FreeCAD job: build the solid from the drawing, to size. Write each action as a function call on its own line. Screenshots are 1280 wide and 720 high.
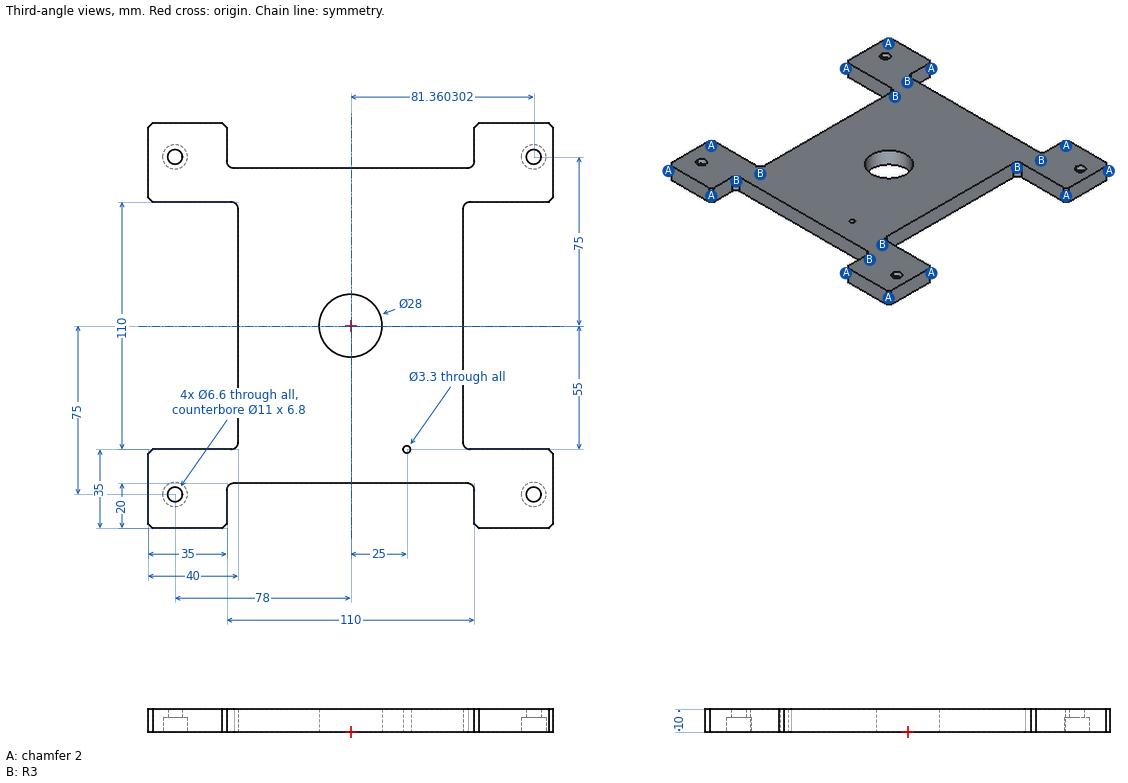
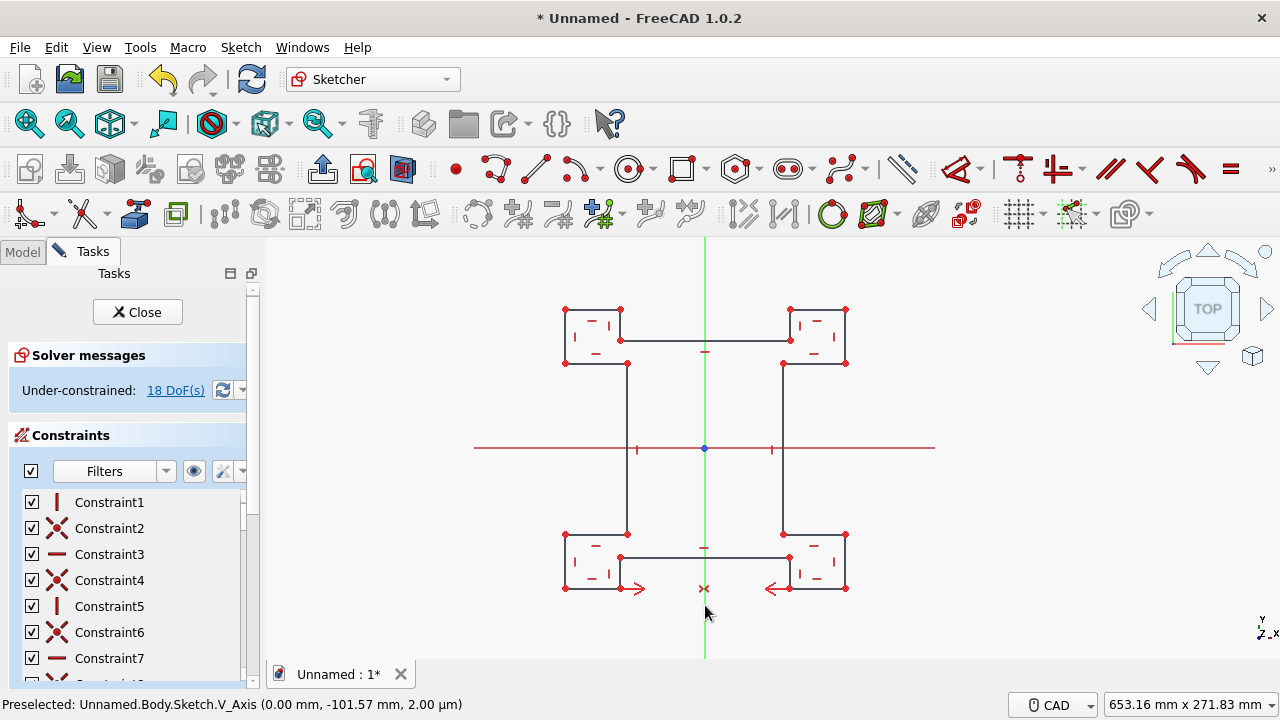
click(565, 535)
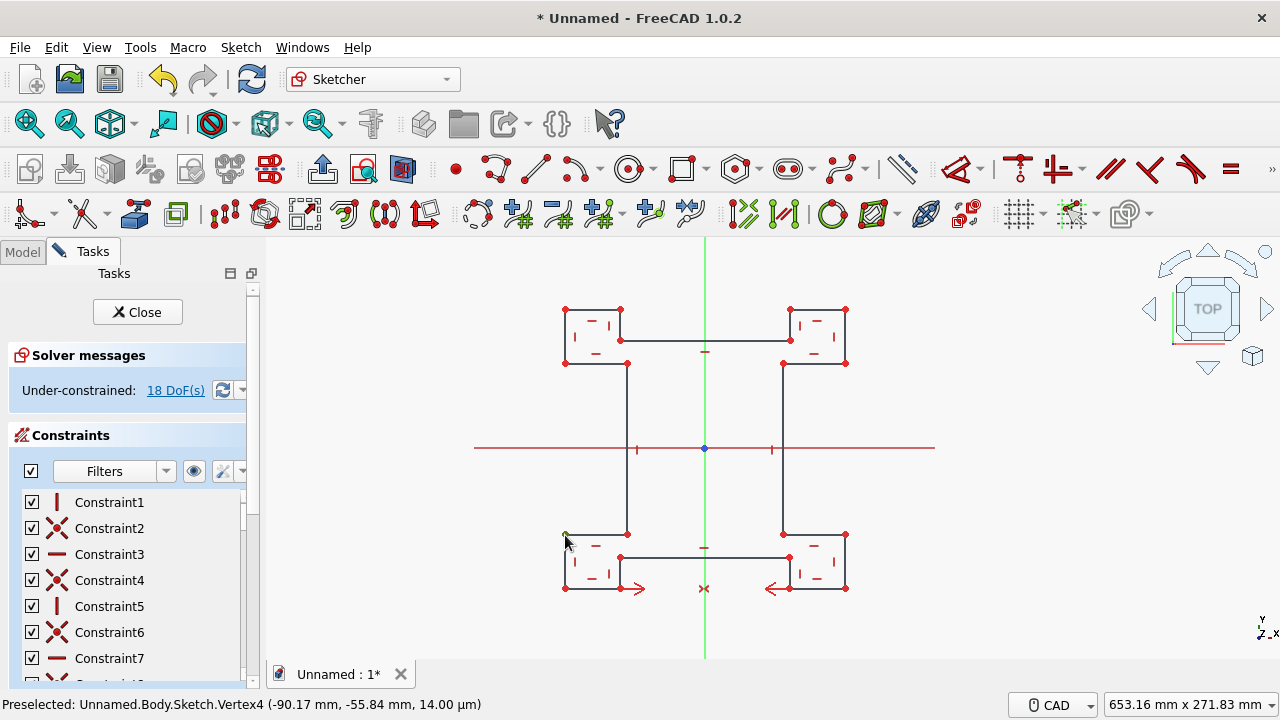
click(845, 535)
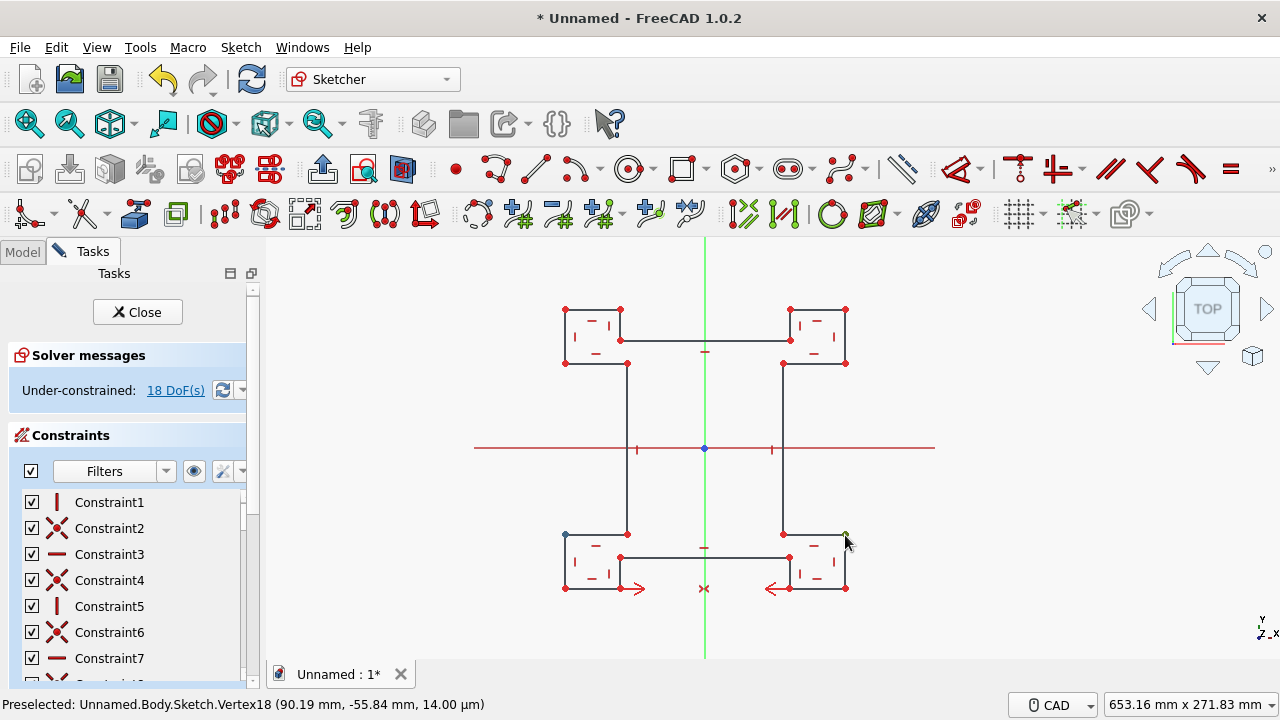
click(705, 605)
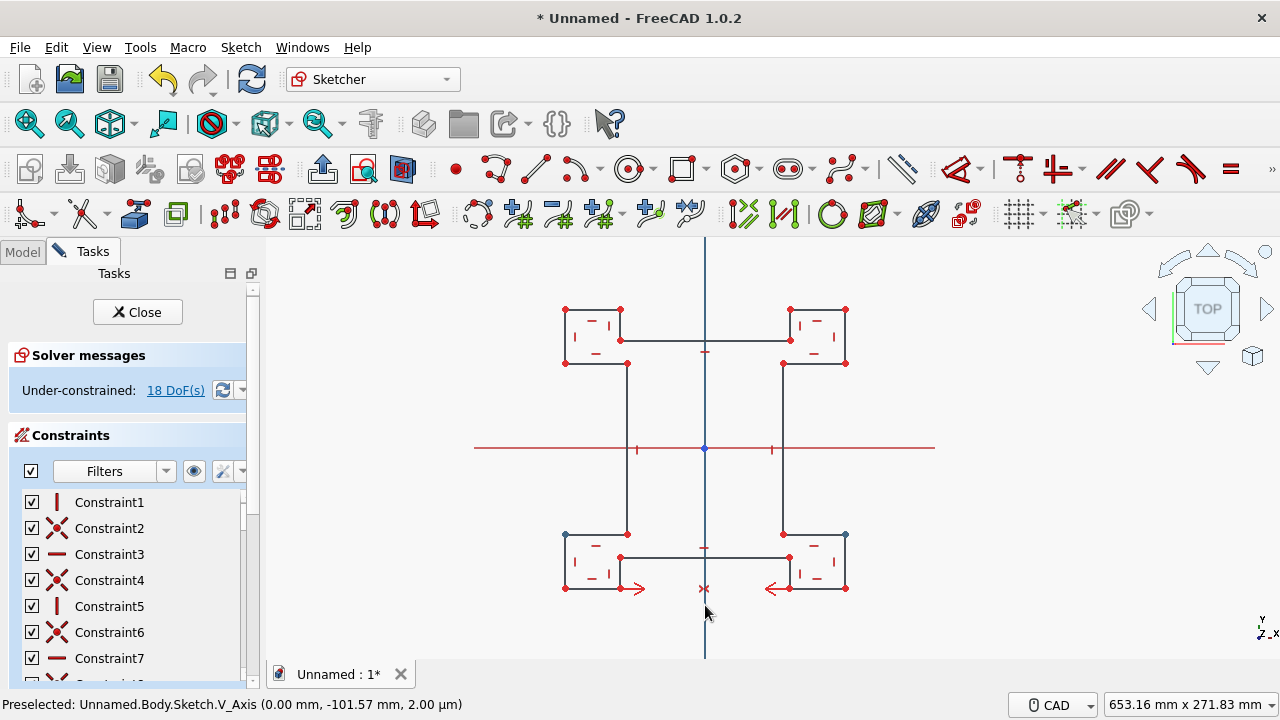
key(s)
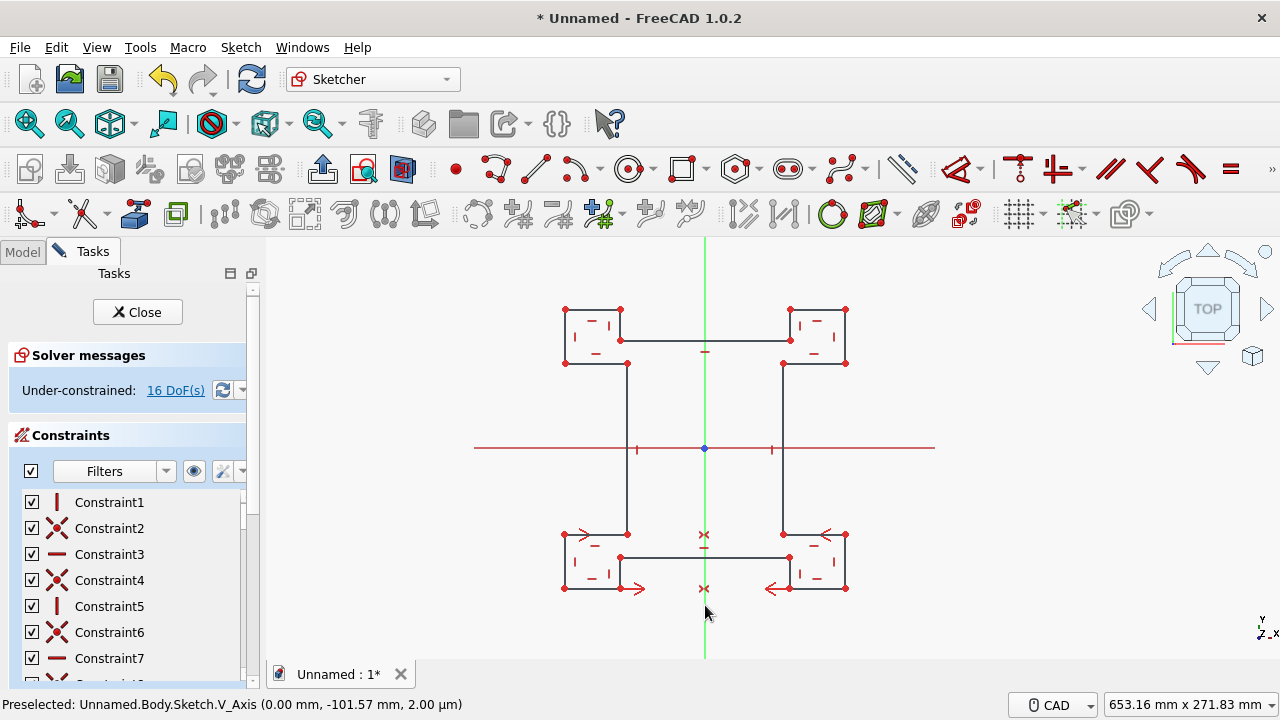
click(627, 364)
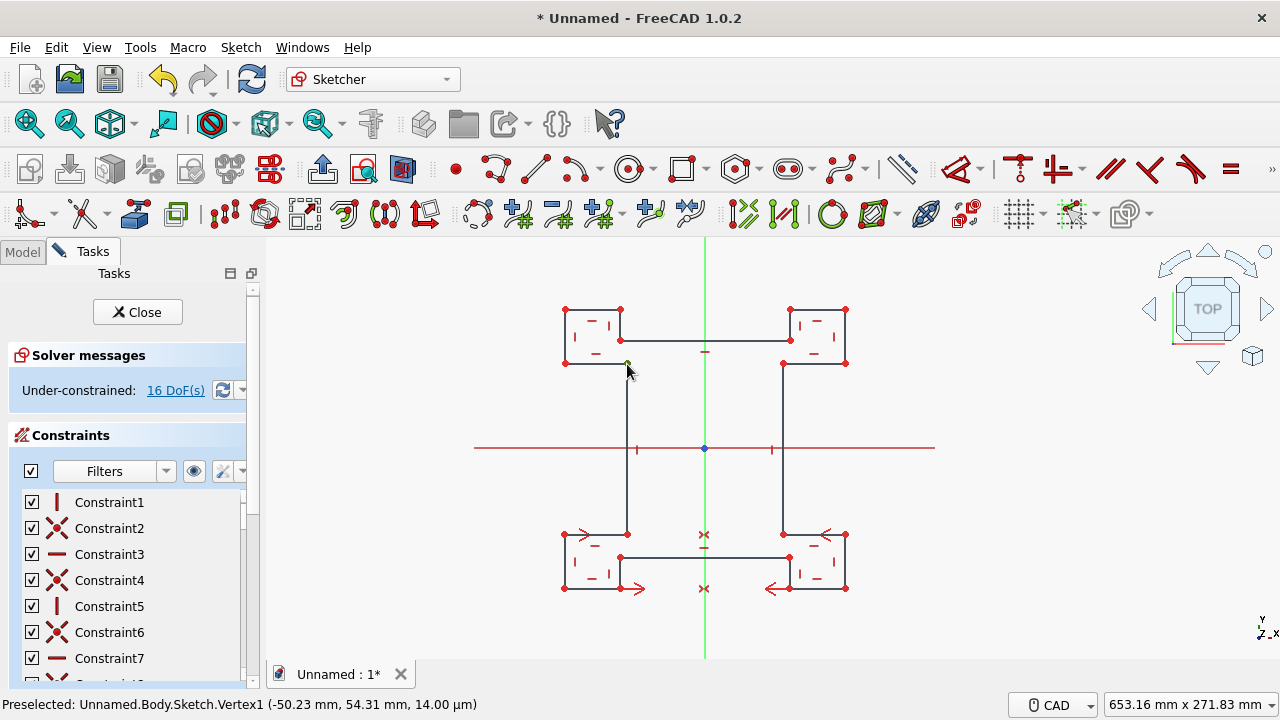
click(783, 364)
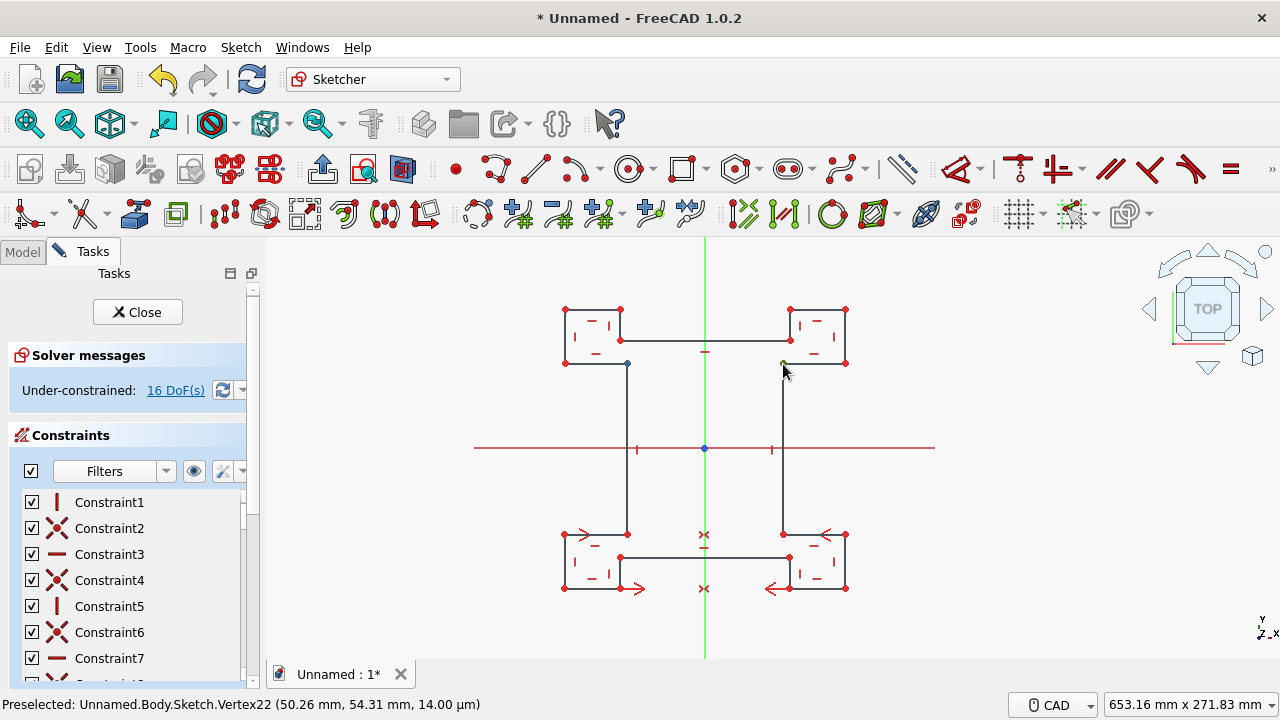
click(705, 605)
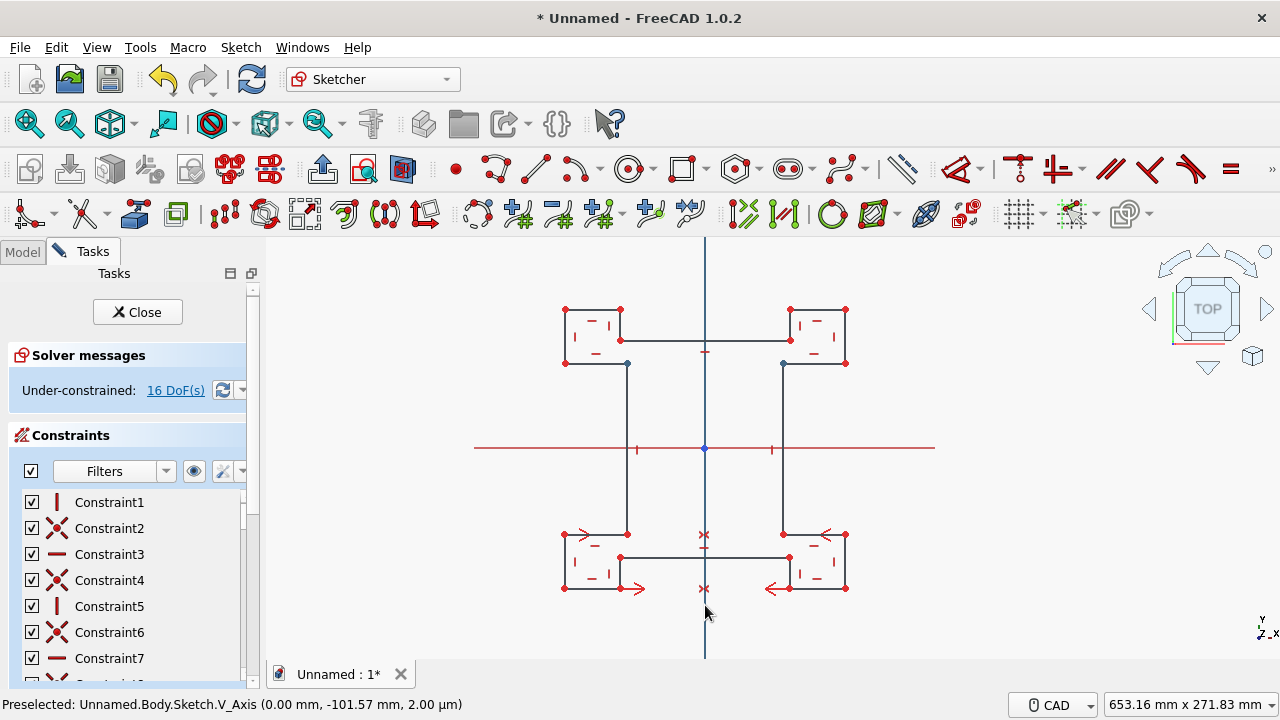
key(s)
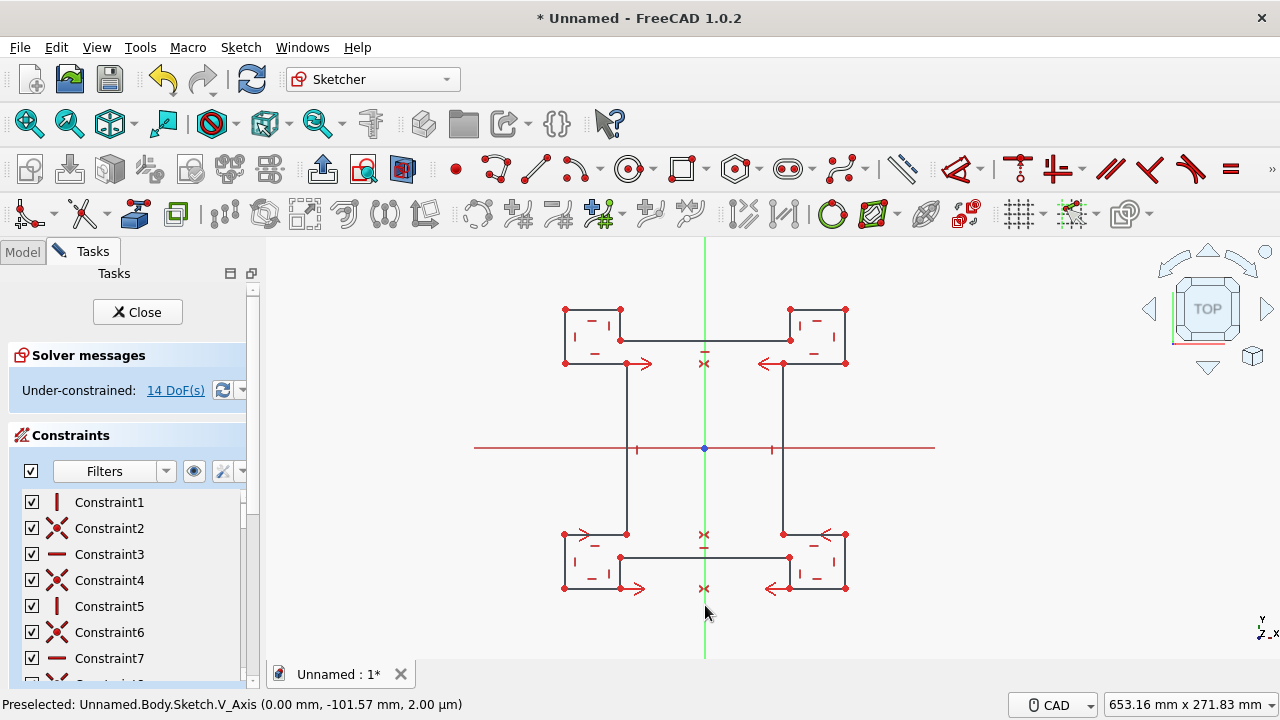
click(845, 535)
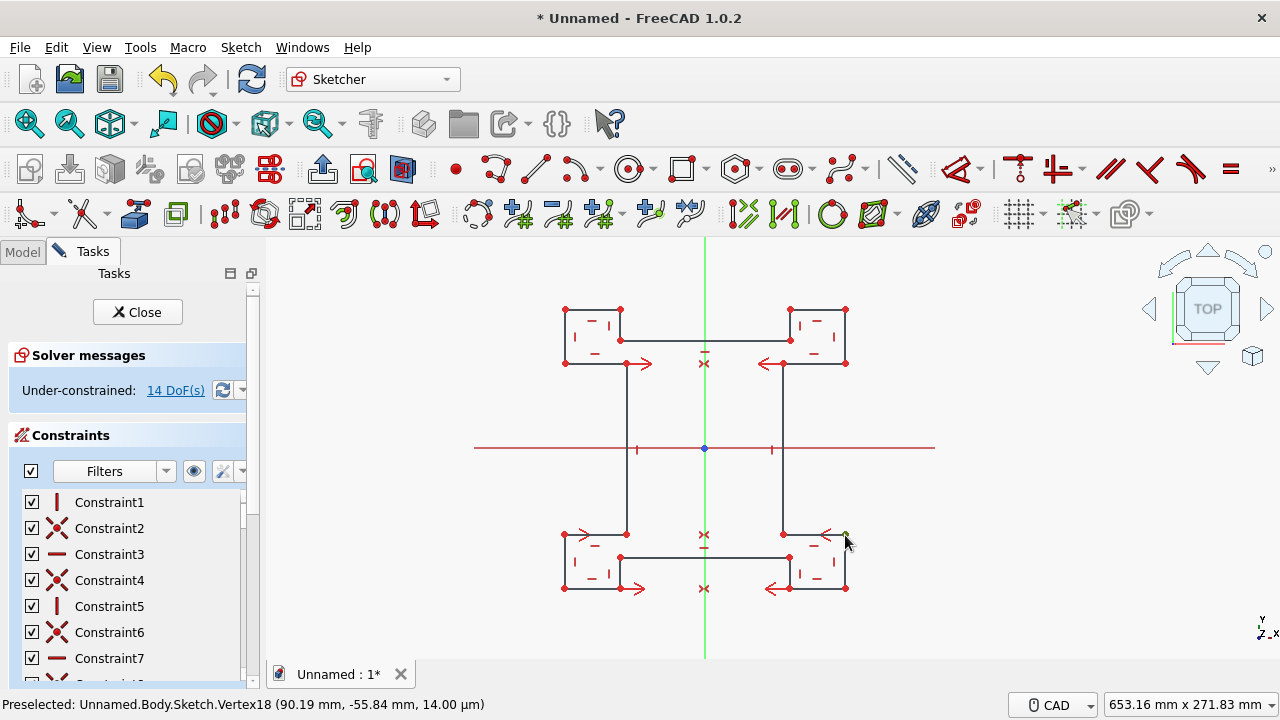
click(845, 364)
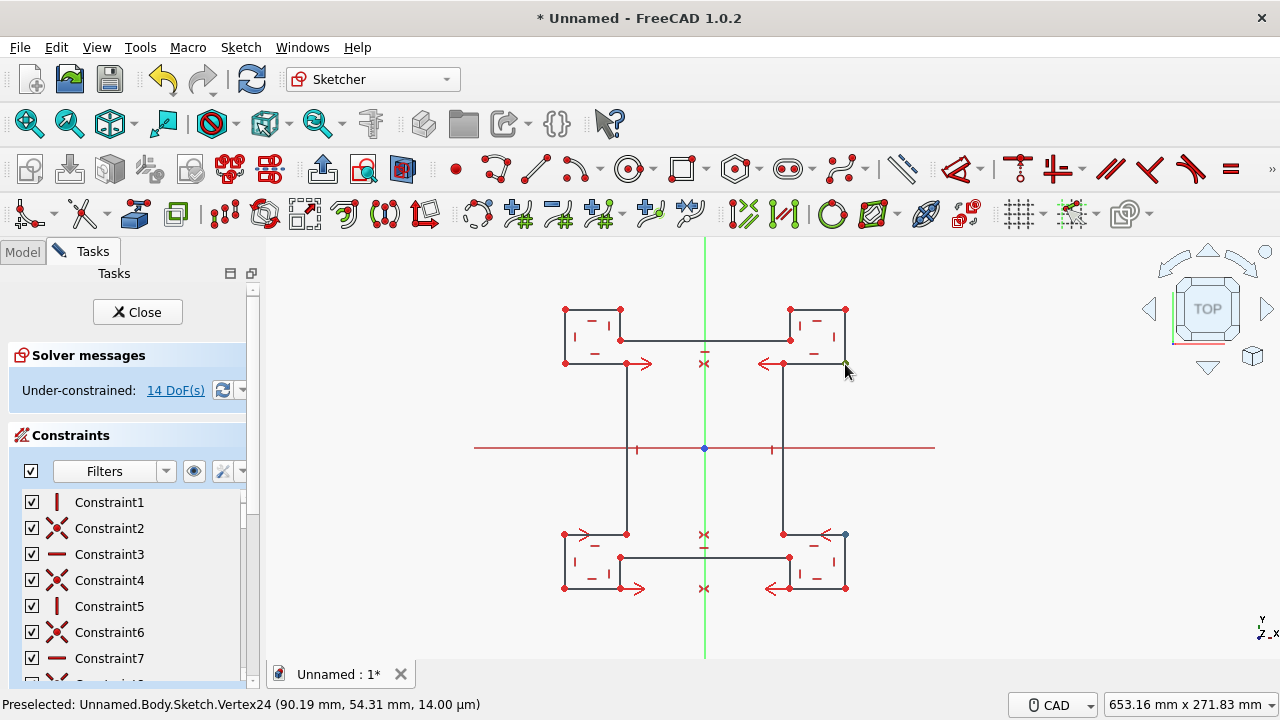
click(470, 448)